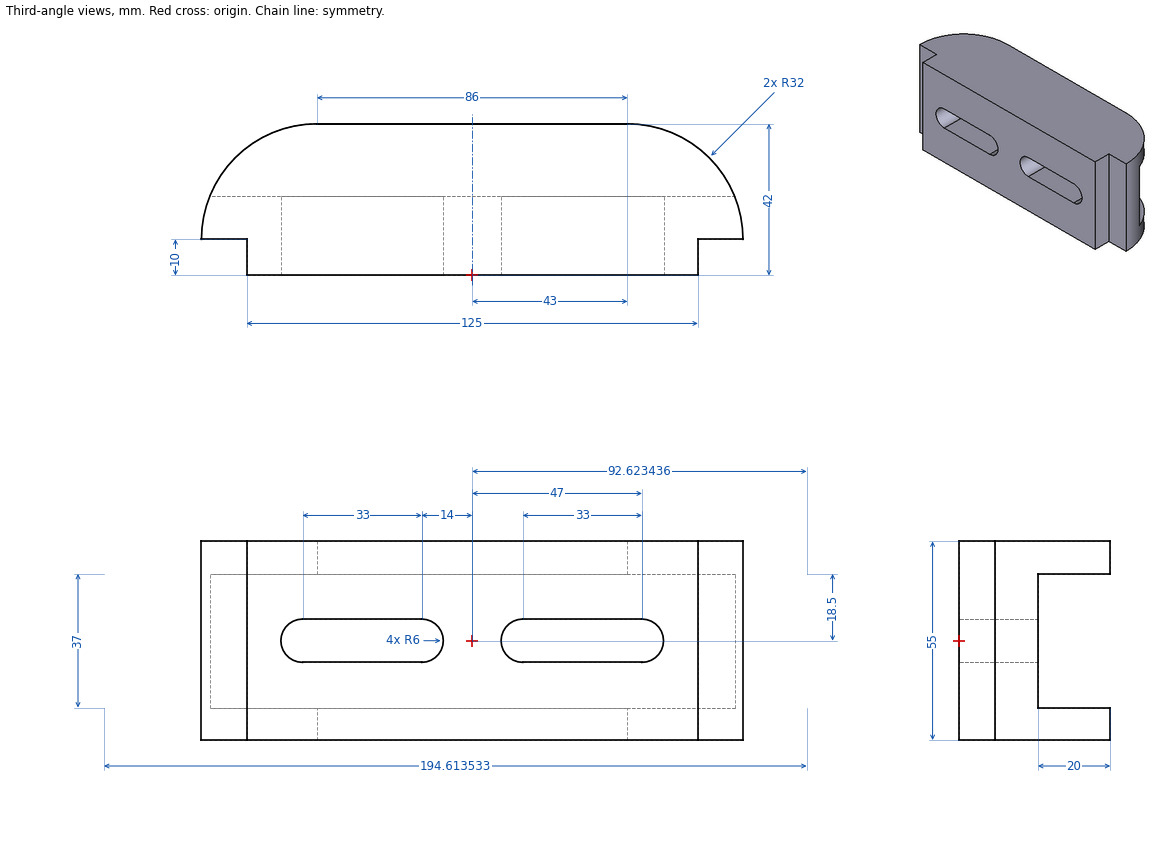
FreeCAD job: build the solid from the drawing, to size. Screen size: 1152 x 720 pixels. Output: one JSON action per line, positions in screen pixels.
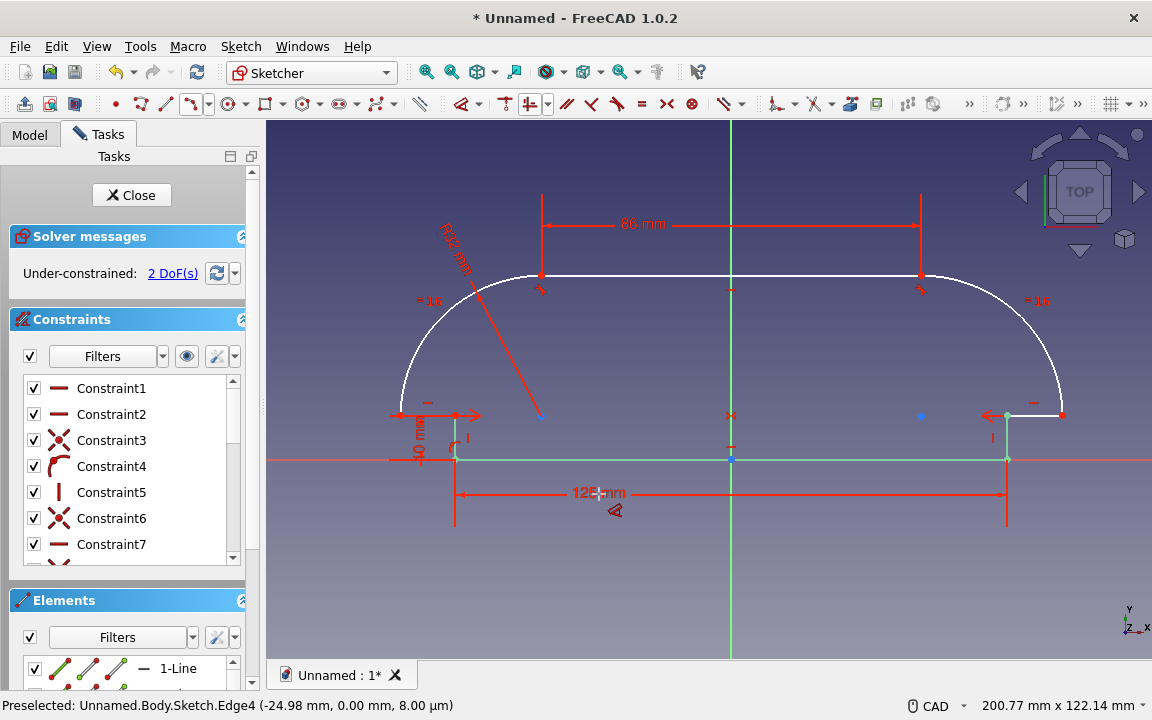
{"action": "left_click", "coordinate": [921, 276]}
{"action": "left_click", "coordinate": [826, 494]}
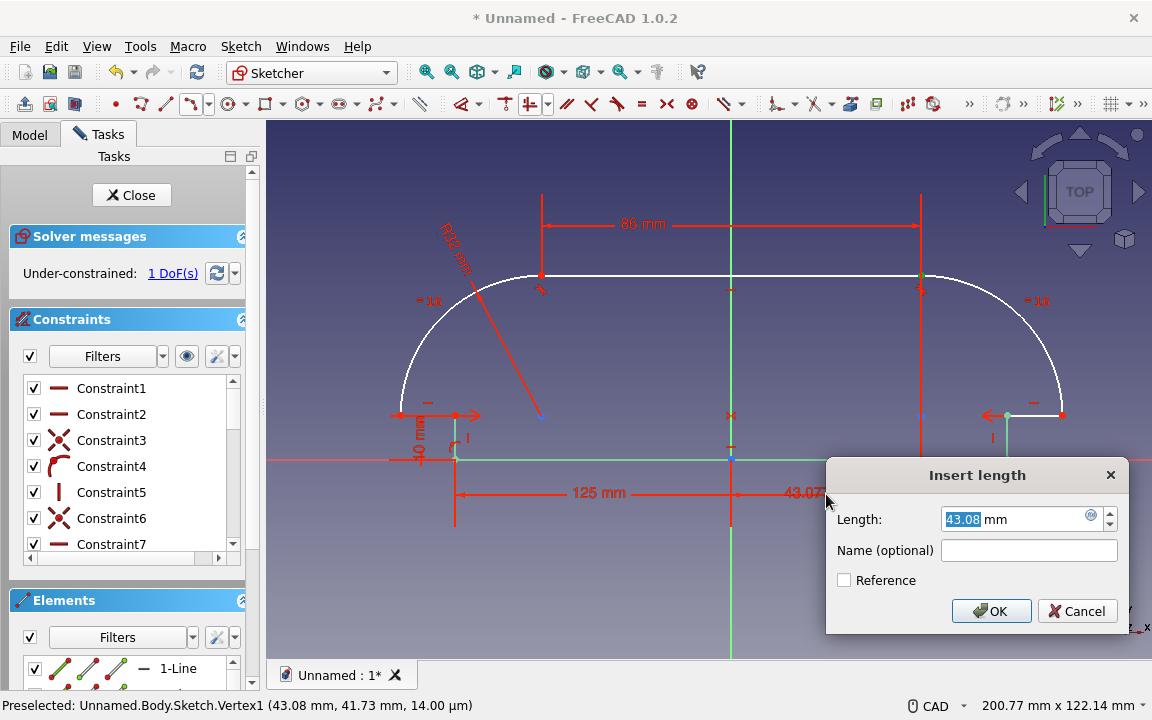
{"action": "type", "text": "43"}
{"action": "key", "text": "Return"}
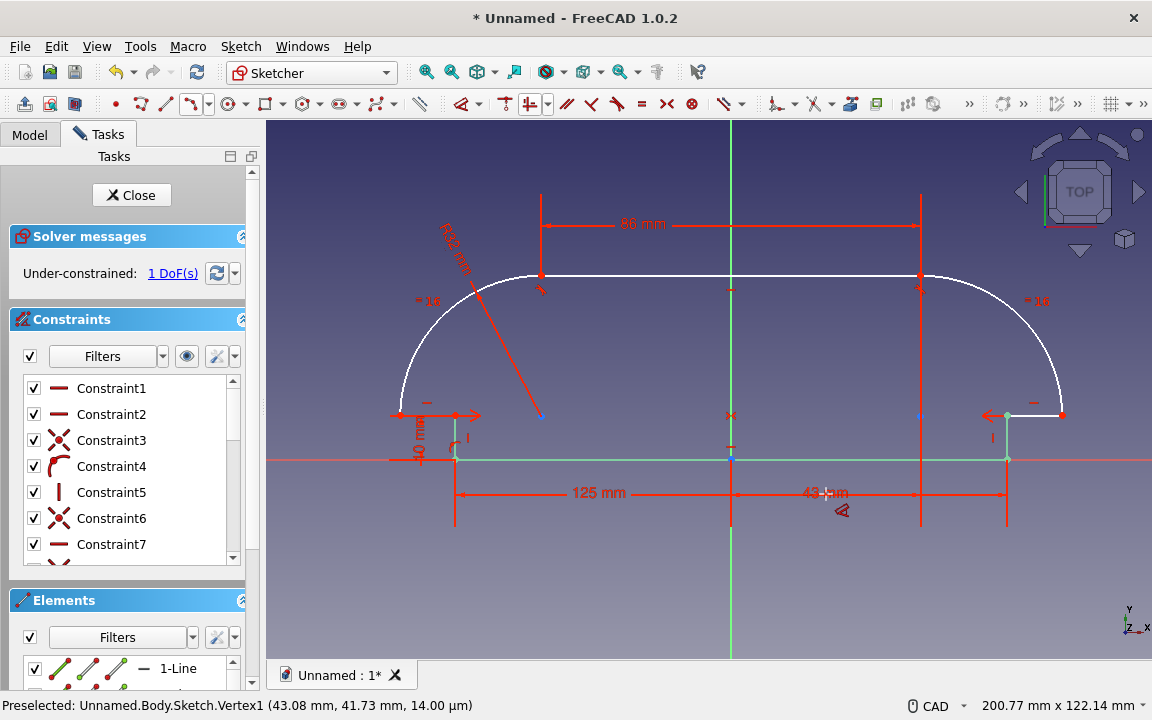
{"action": "left_click", "coordinate": [921, 276]}
{"action": "left_click", "coordinate": [955, 368]}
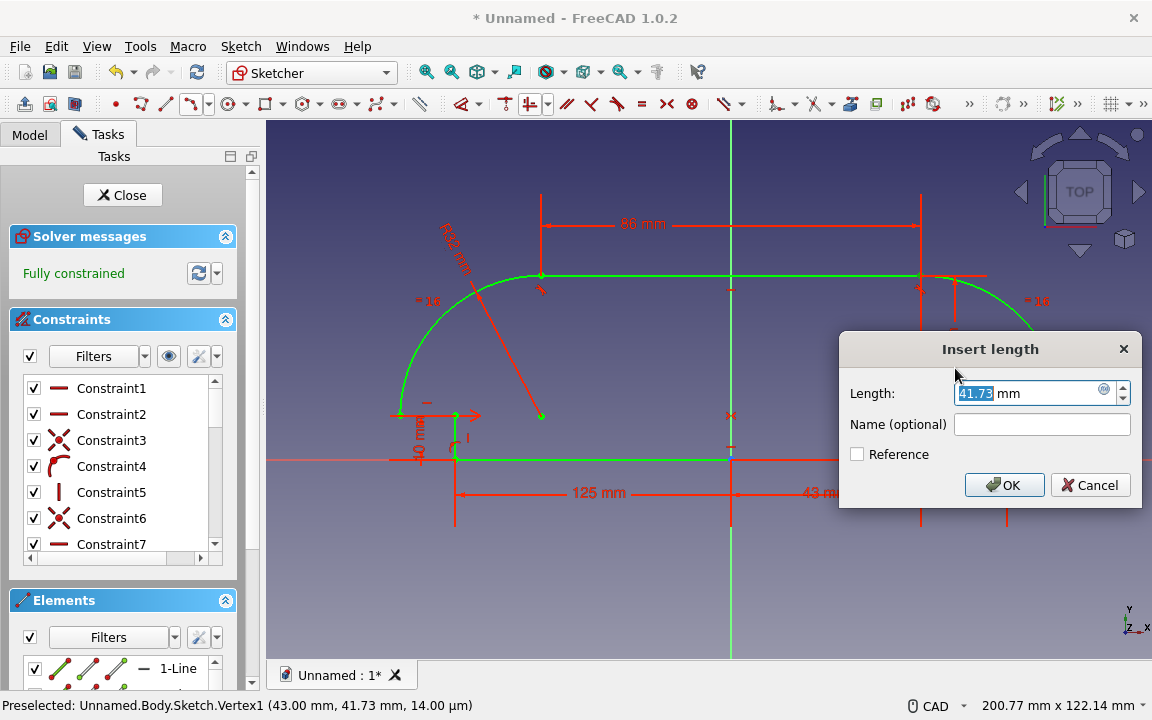
{"action": "type", "text": "42"}
{"action": "key", "text": "Return"}
{"action": "key", "text": "Escape"}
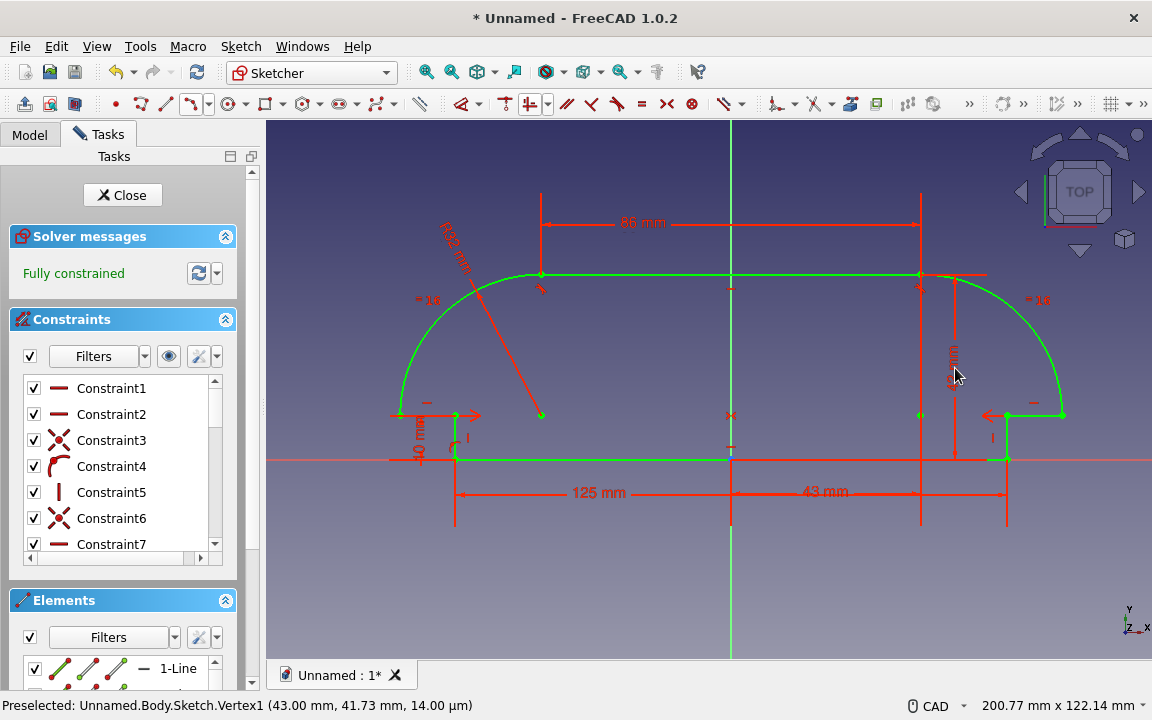
{"action": "left_click", "coordinate": [123, 195]}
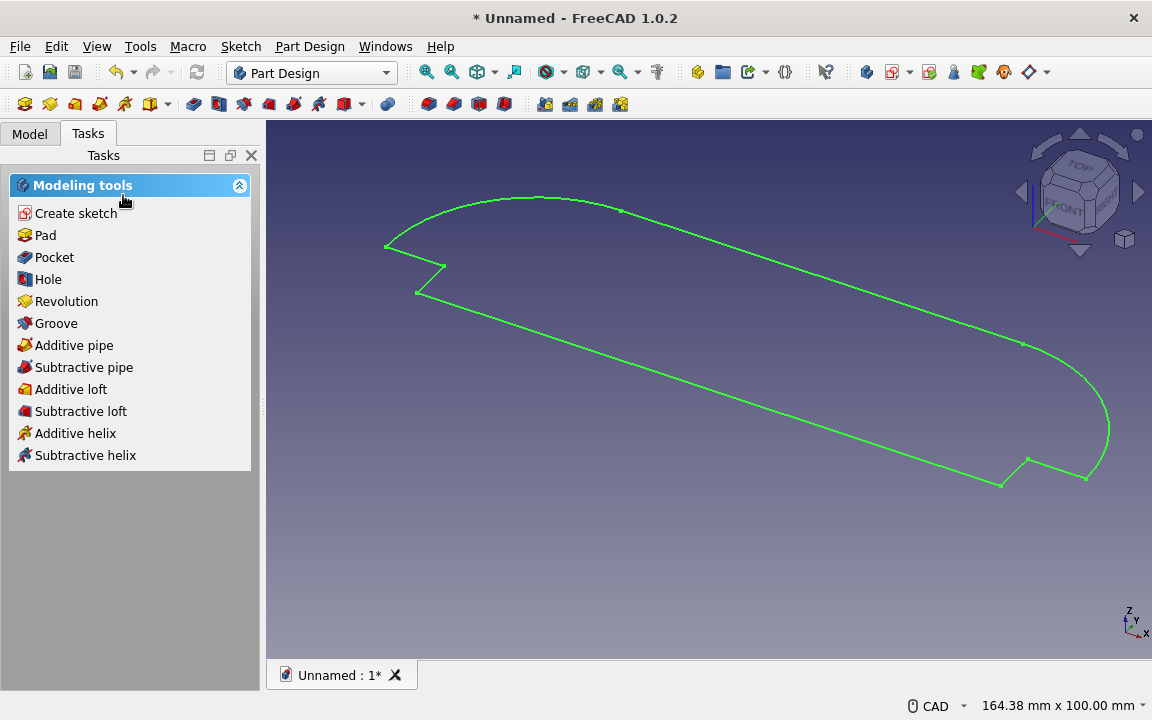
{"action": "left_click", "coordinate": [25, 104]}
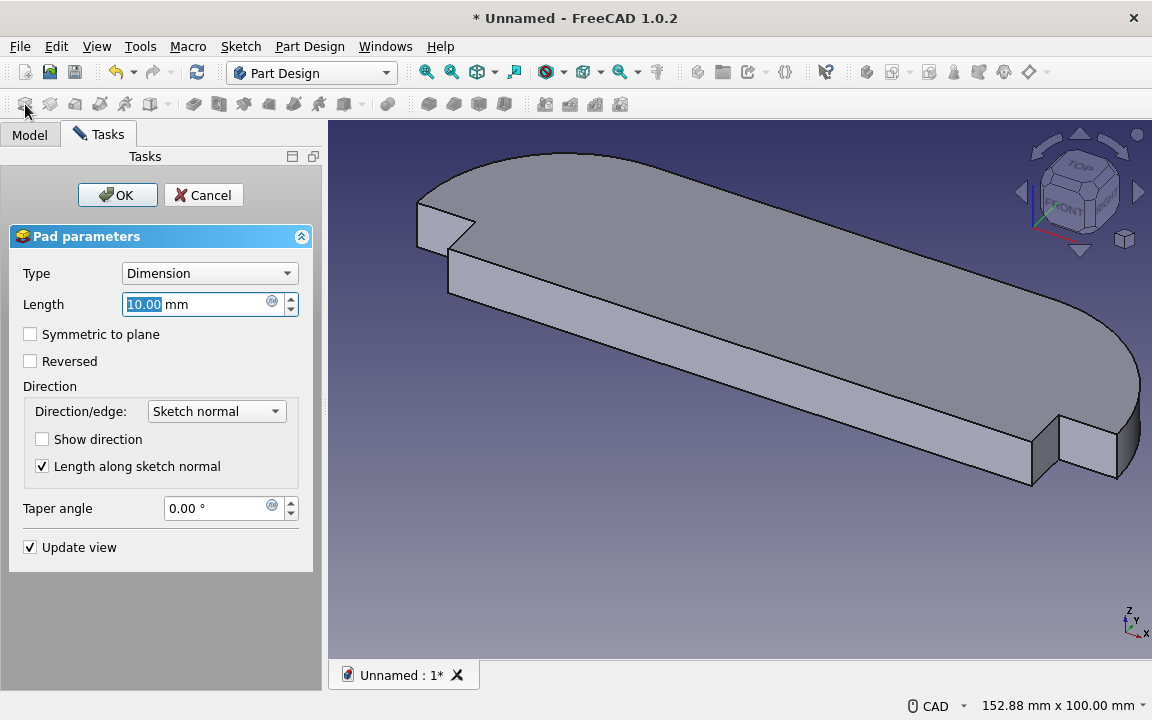
{"action": "type", "text": "55"}
{"action": "key", "text": "Tab"}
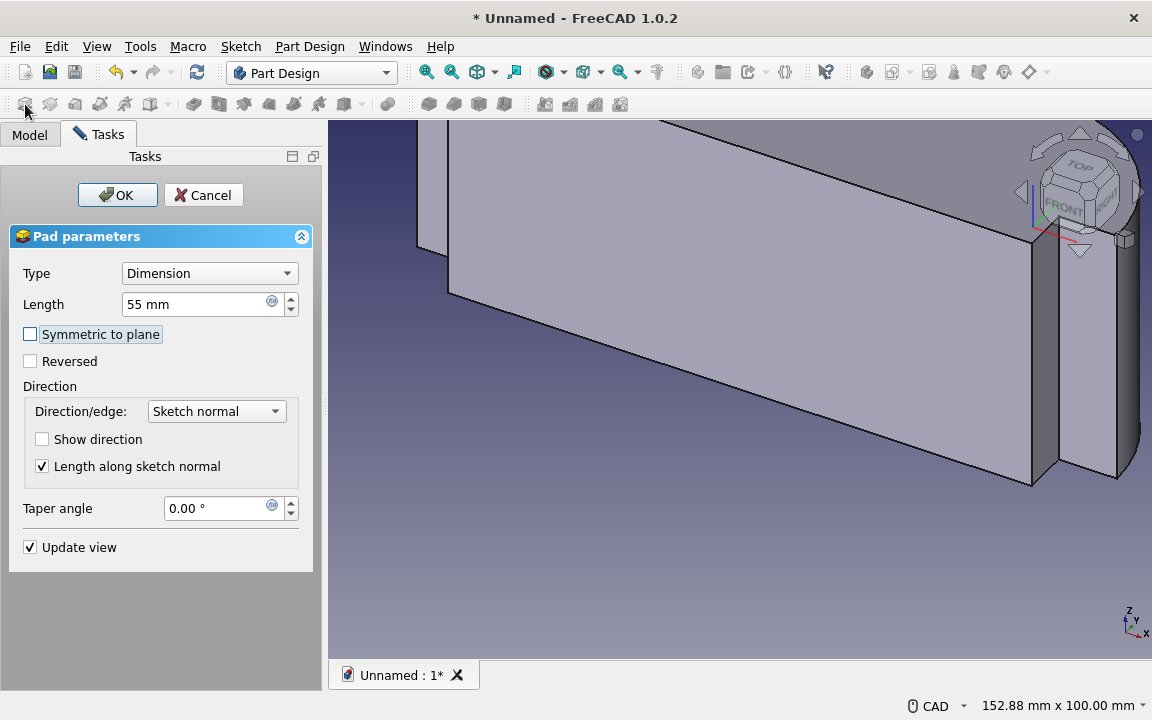
{"action": "left_click", "coordinate": [31, 334]}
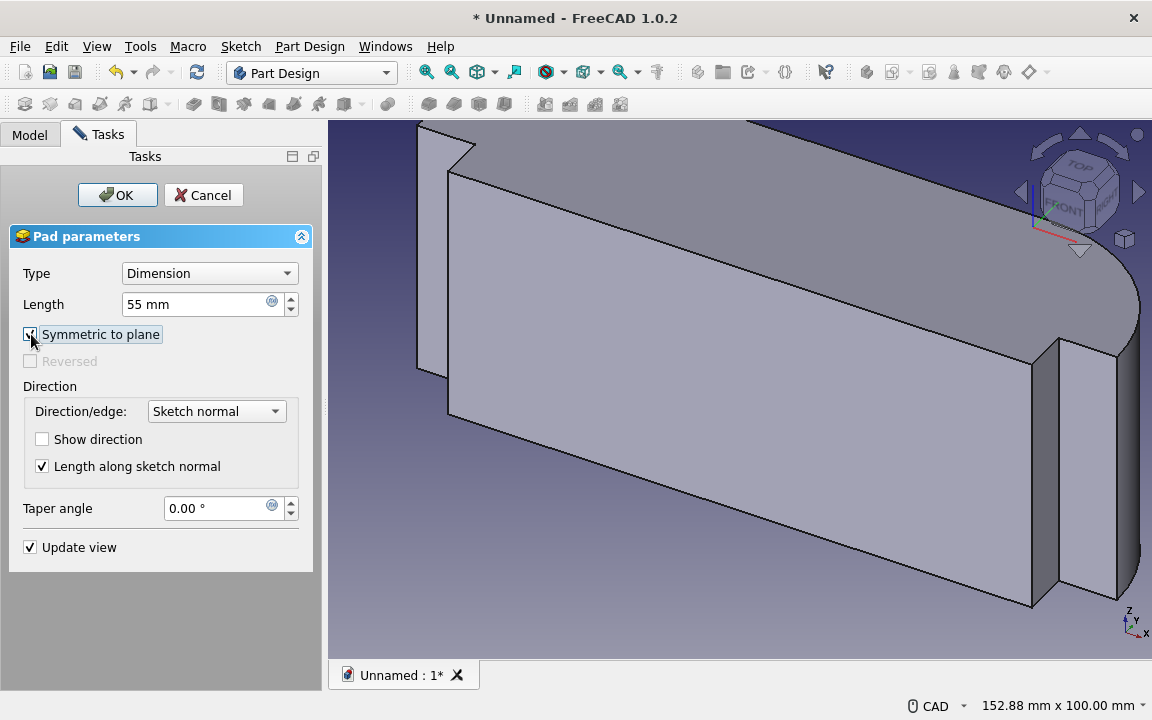
{"action": "left_click", "coordinate": [118, 195]}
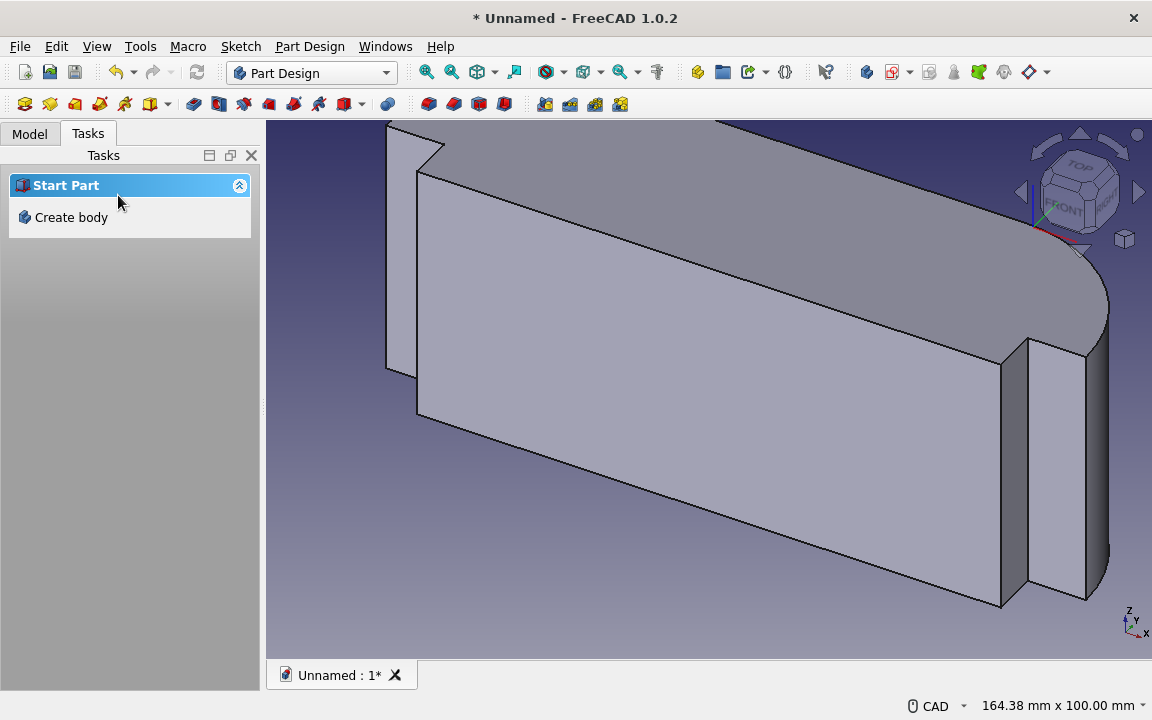
{"action": "left_click", "coordinate": [427, 72]}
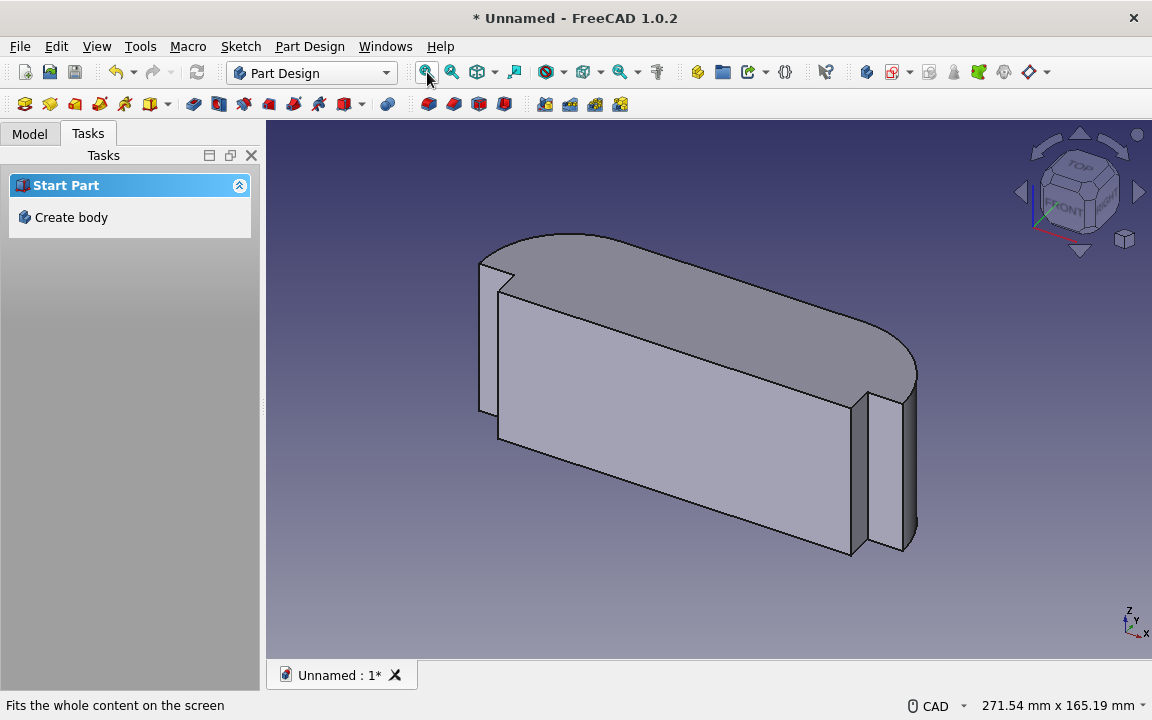
{"action": "key", "text": "4"}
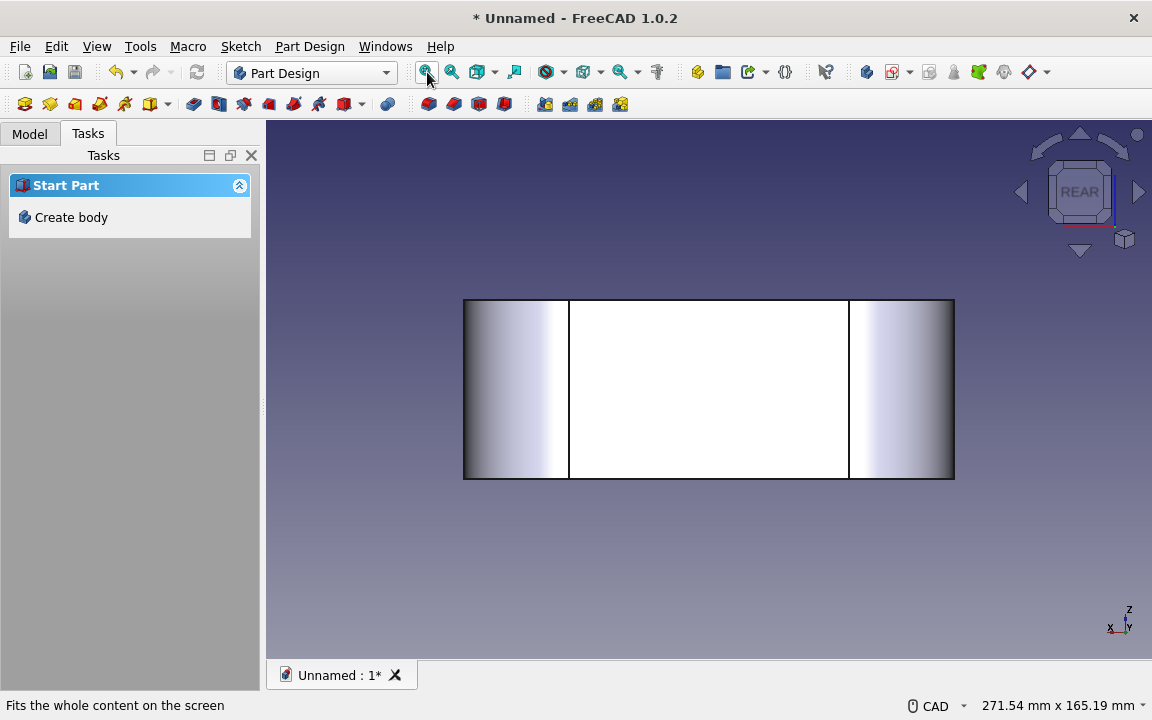
{"action": "left_click", "coordinate": [669, 388]}